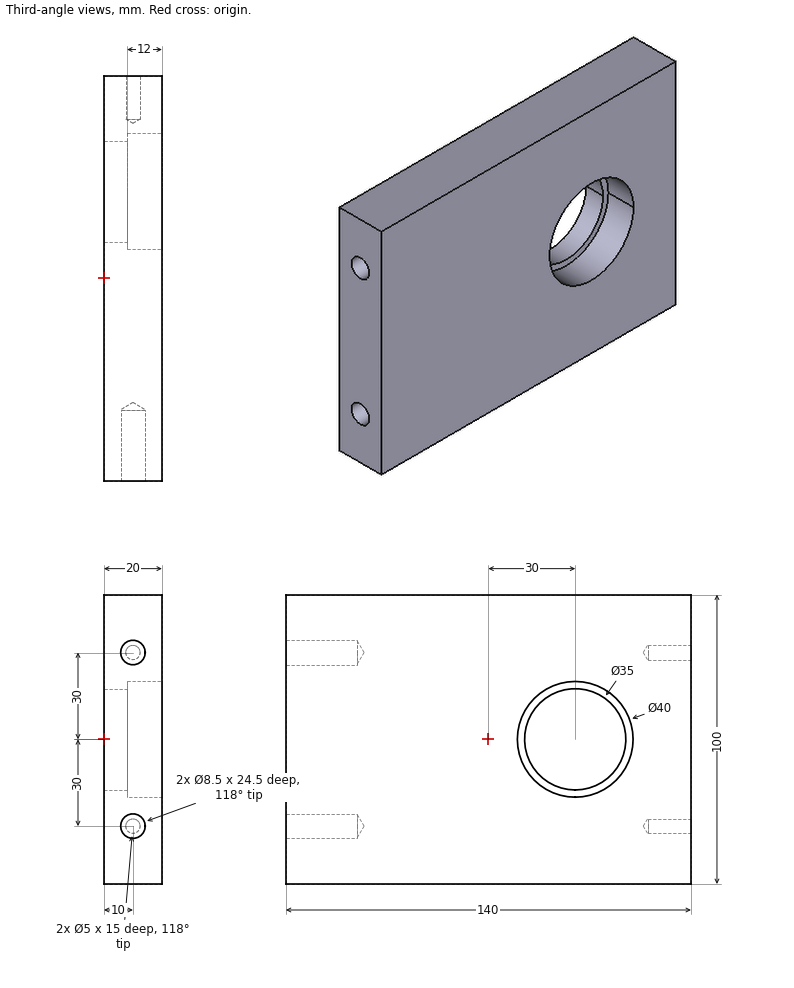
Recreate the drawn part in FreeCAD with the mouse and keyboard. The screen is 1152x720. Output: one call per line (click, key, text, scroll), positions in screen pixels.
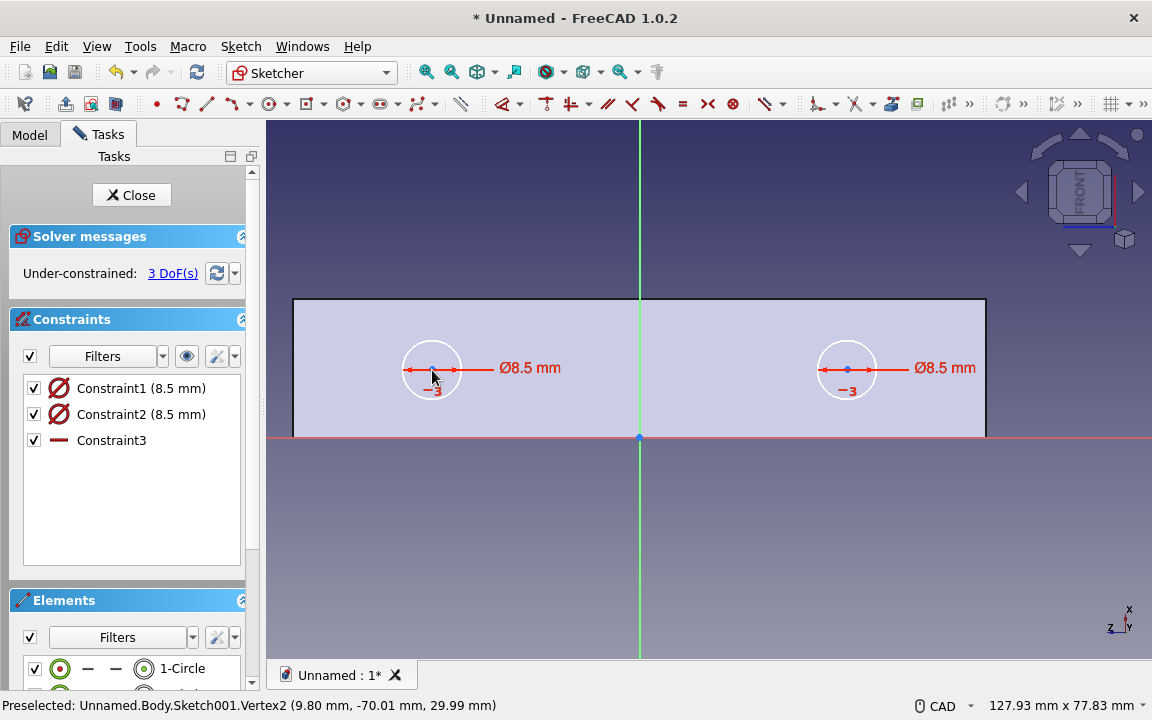
click(502, 104)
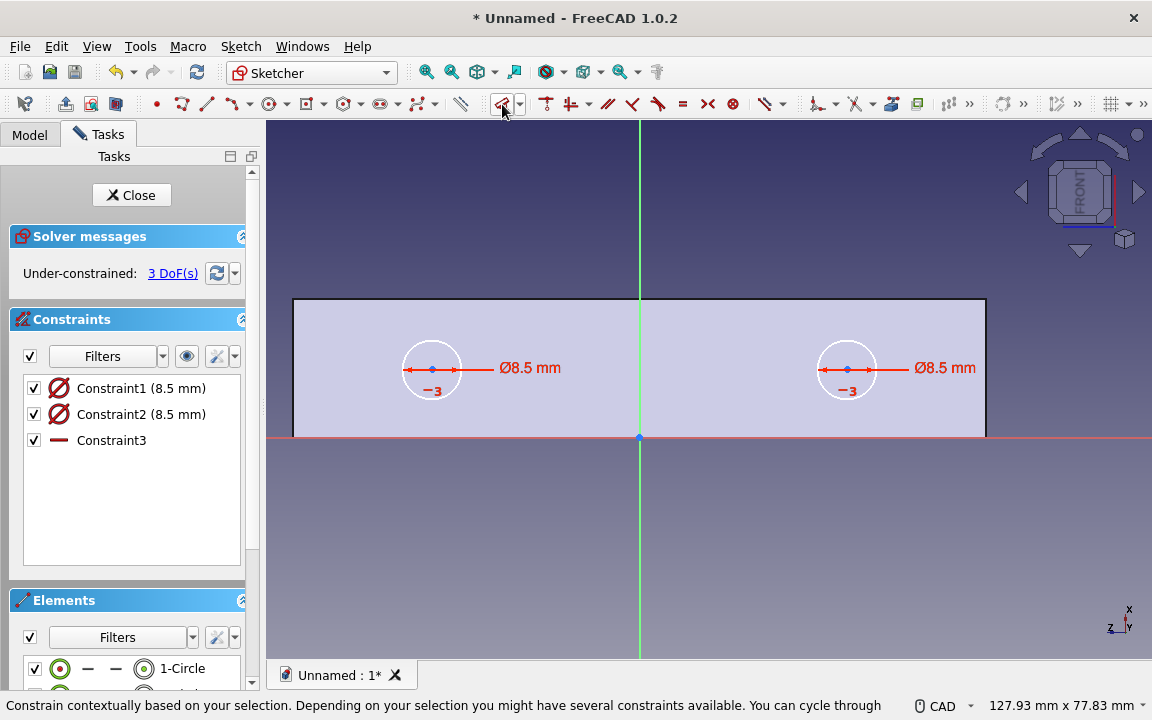
click(847, 370)
click(743, 472)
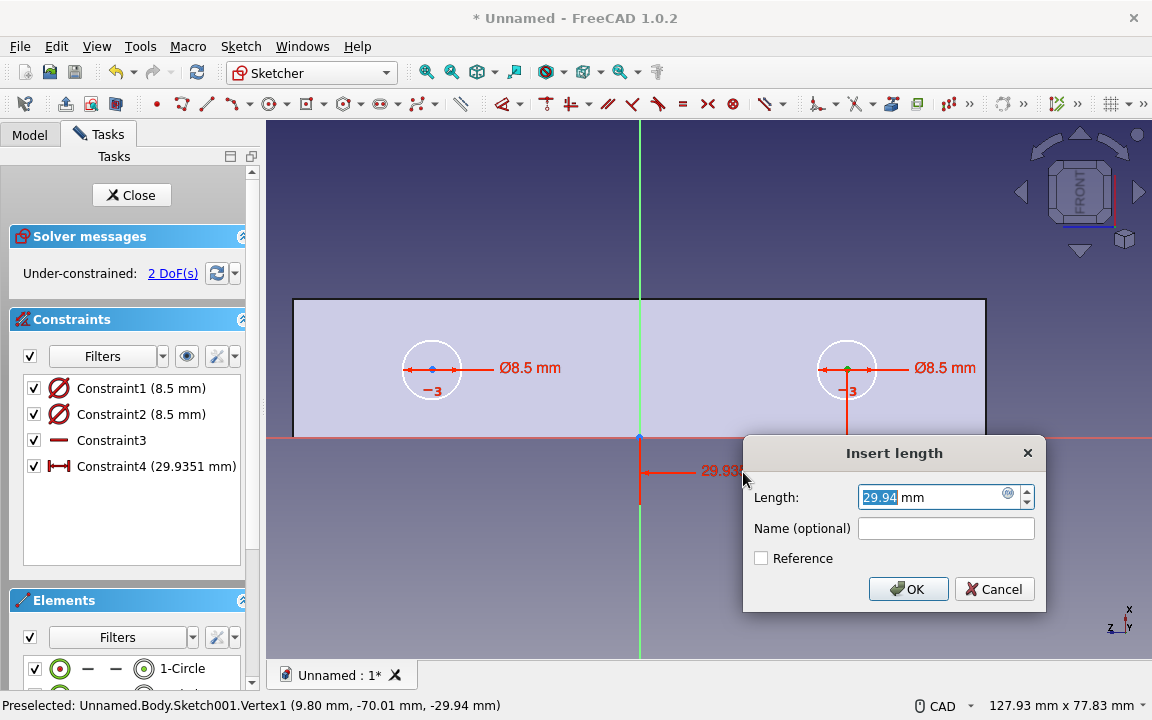
text(30)
key(Return)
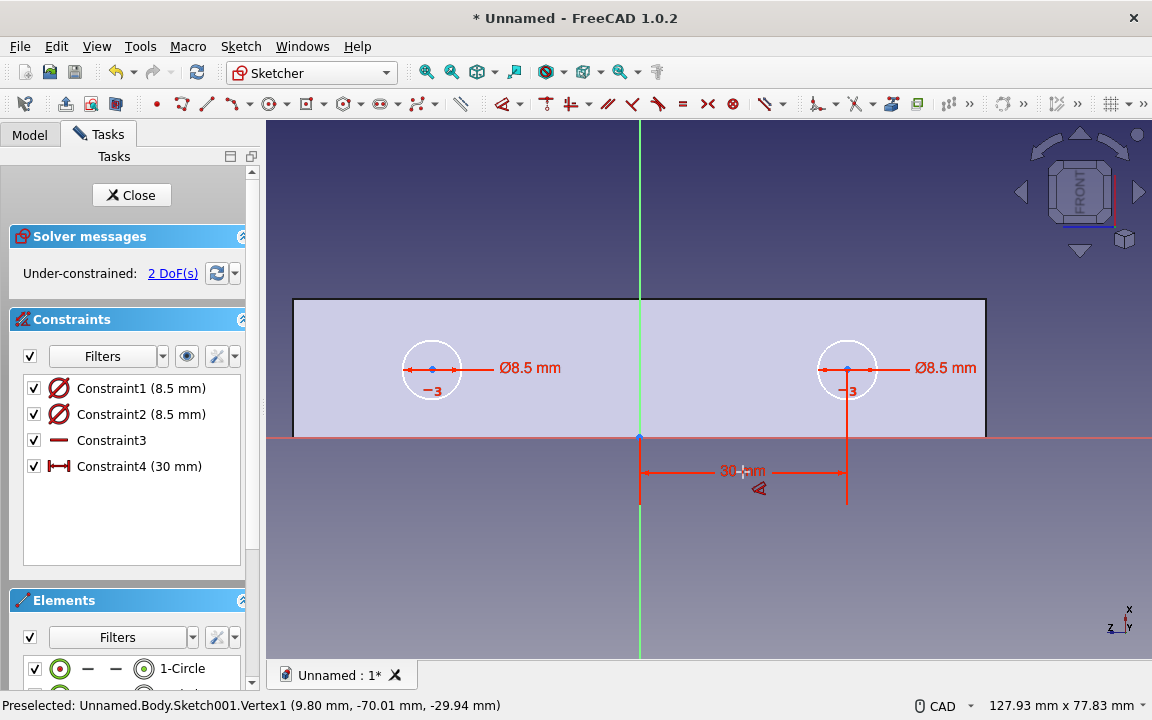
click(847, 370)
click(881, 404)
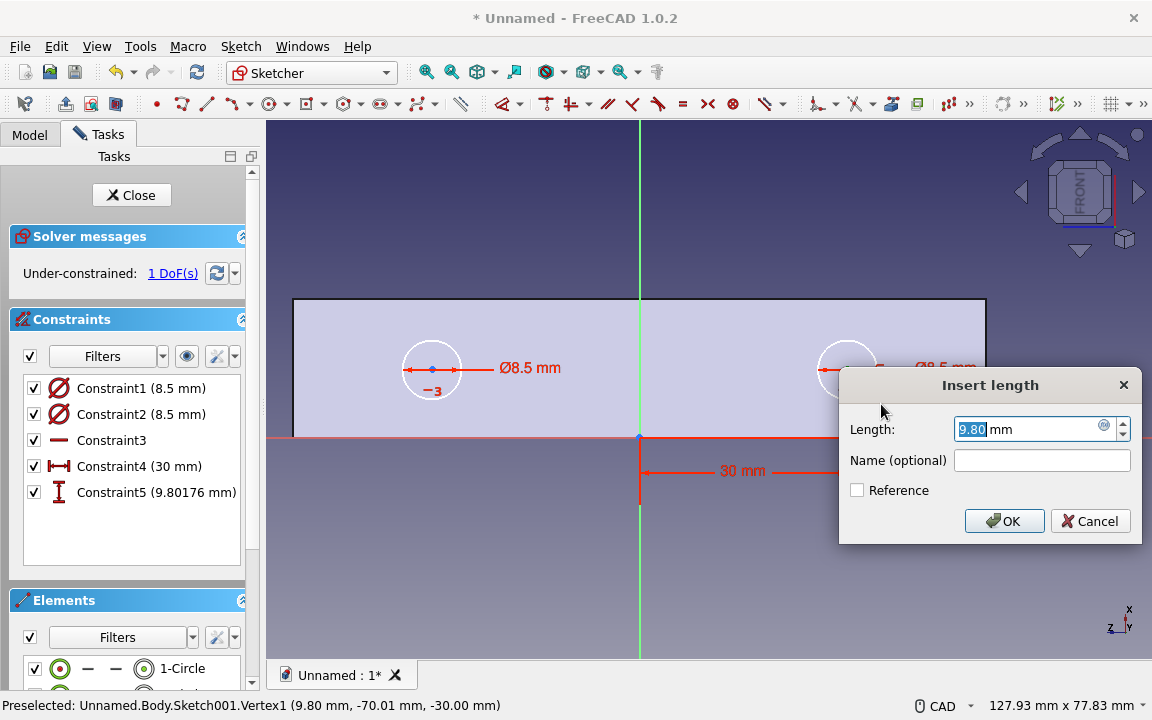
text(10)
key(Return)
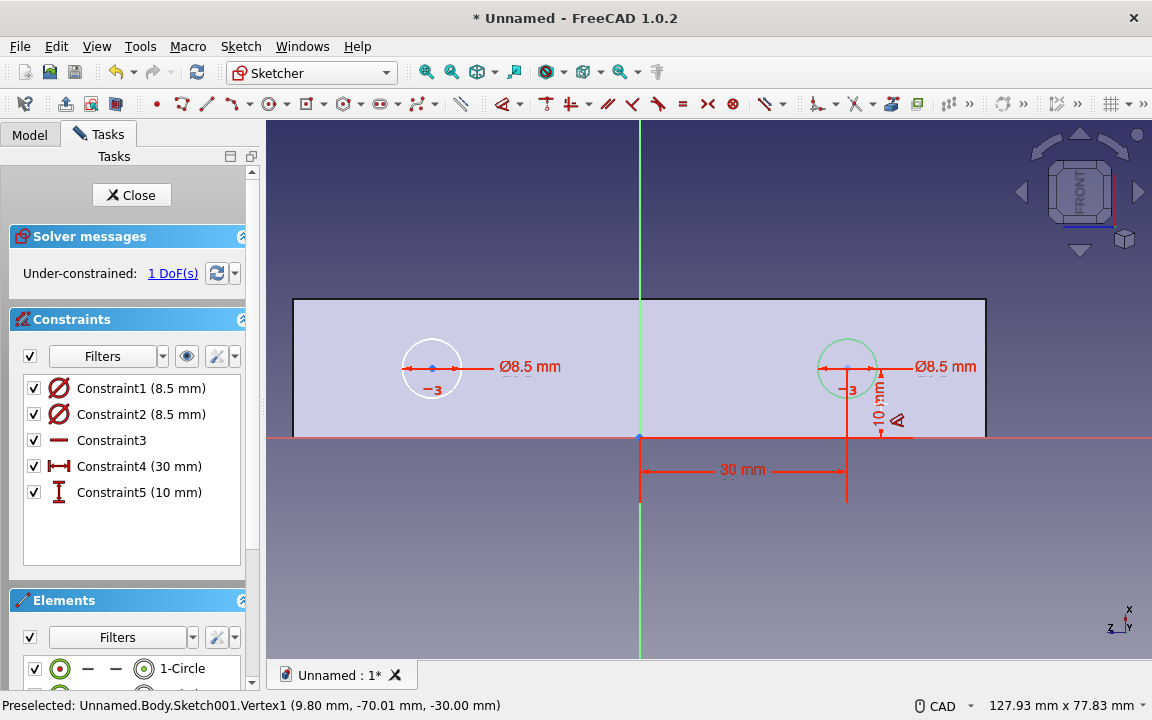
click(432, 369)
click(536, 472)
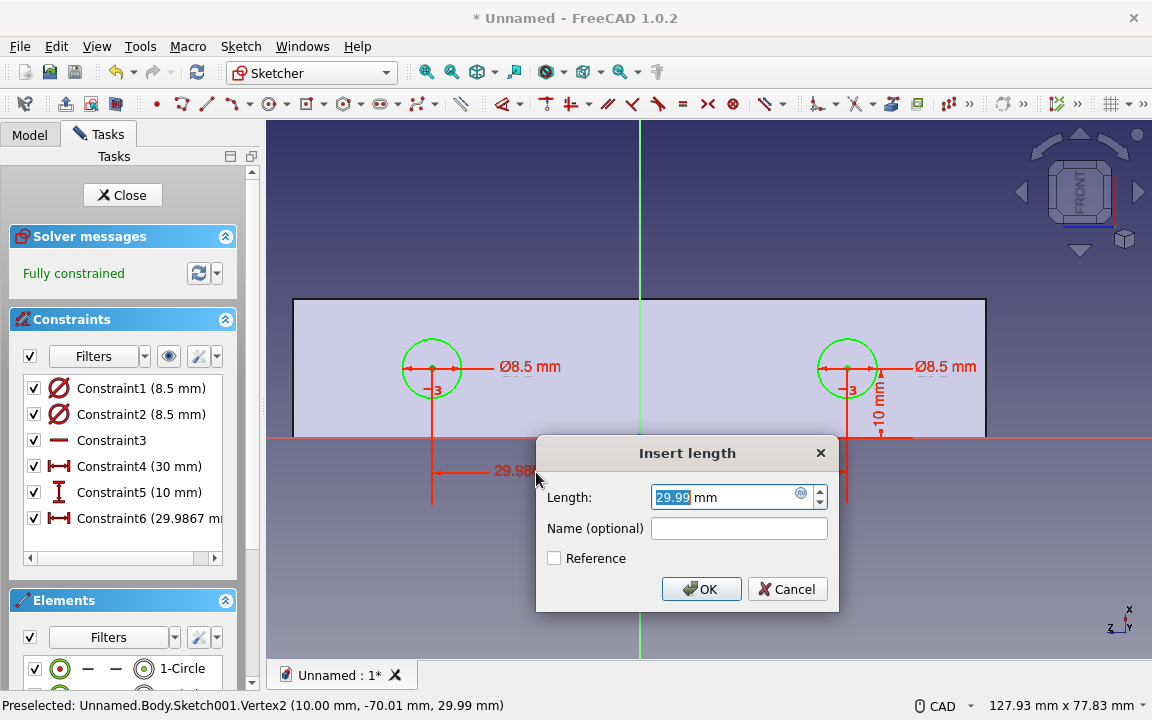
text(30)
key(Return)
key(Escape)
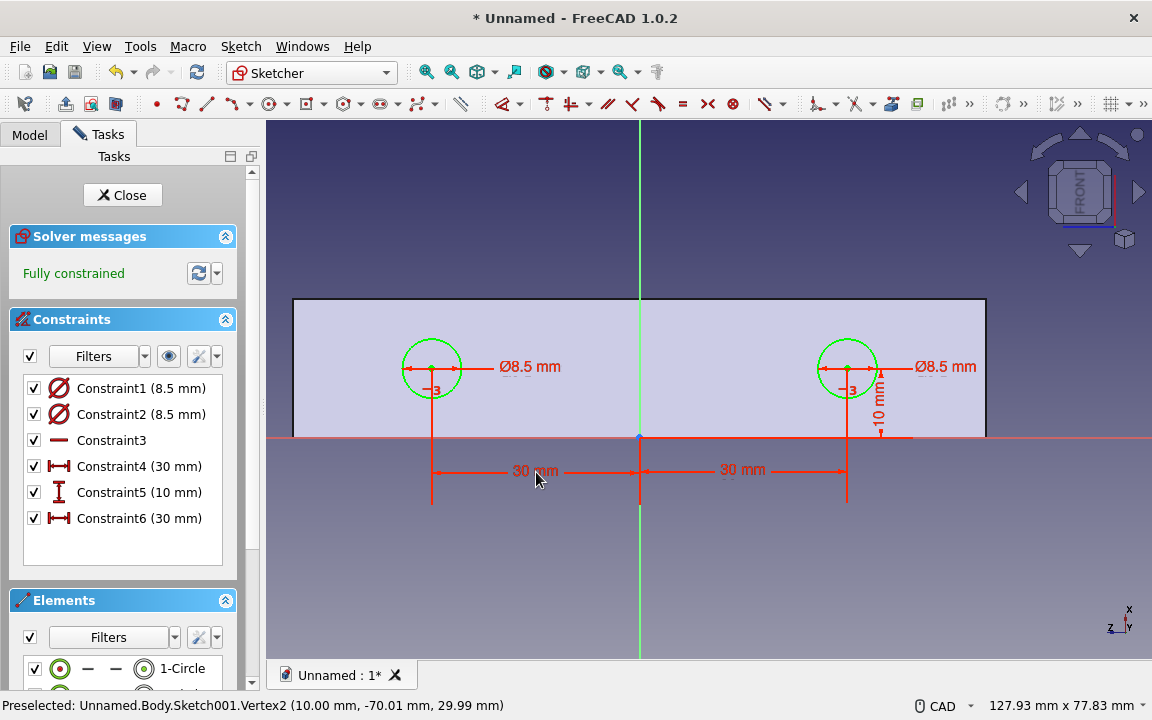
click(123, 195)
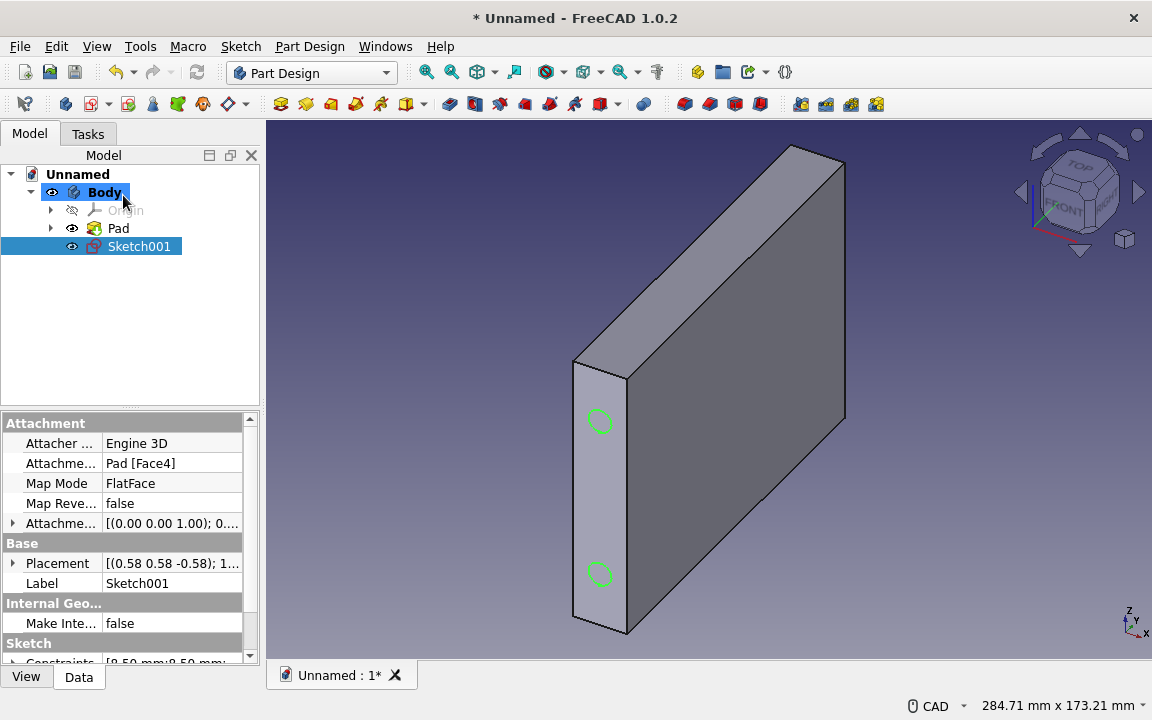
click(475, 104)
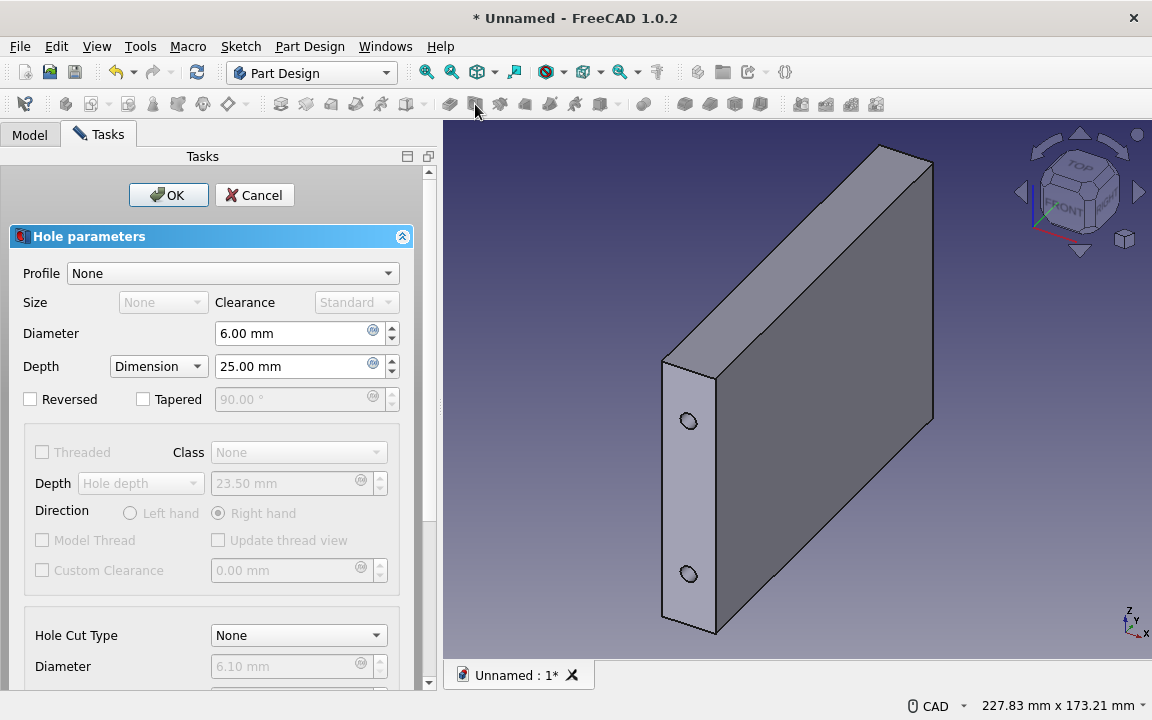
triple_click(300, 334)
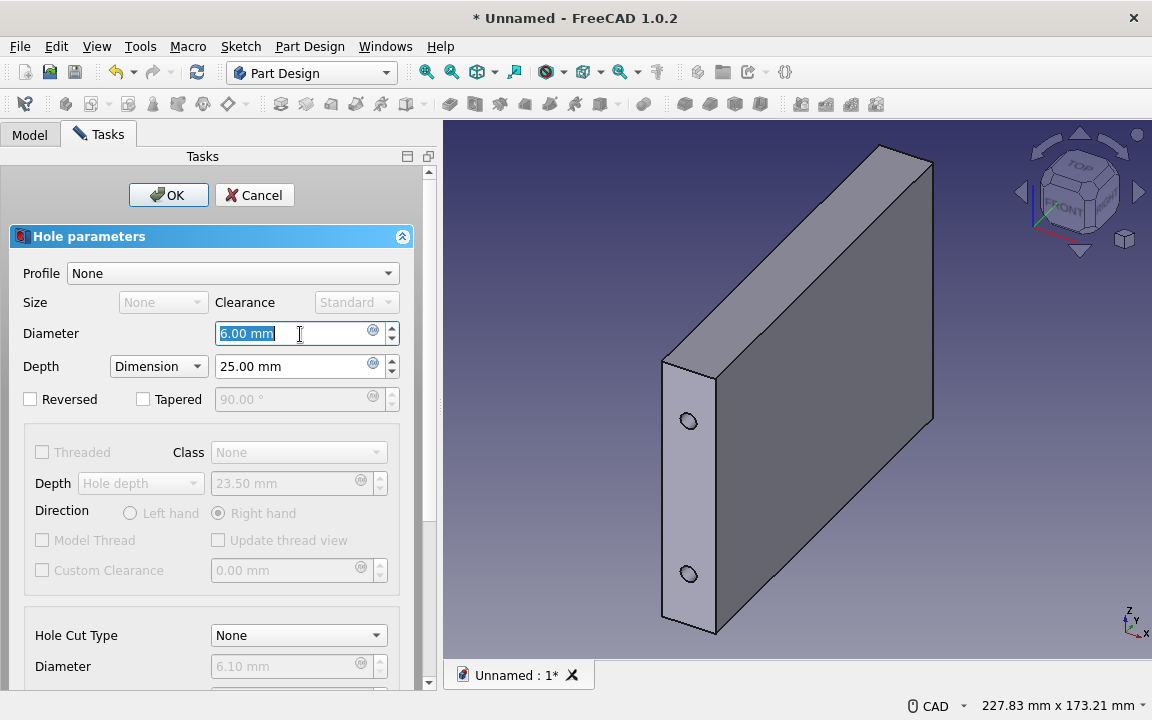
text(8.5)
key(Tab)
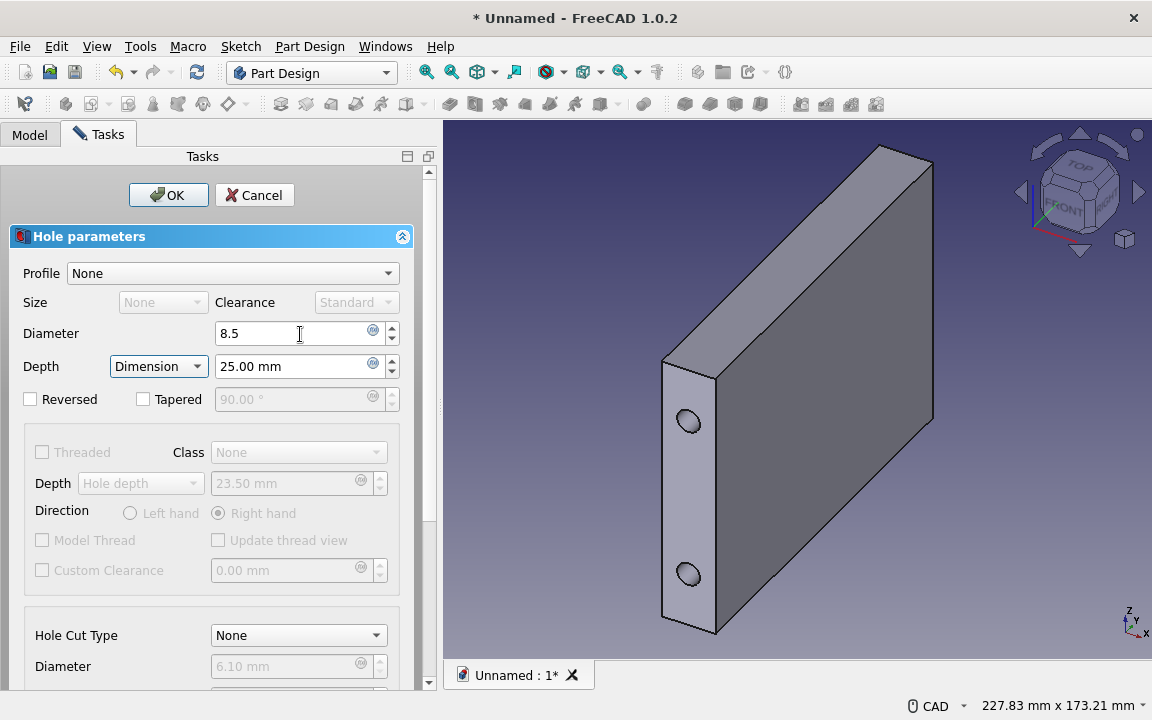
triple_click(300, 366)